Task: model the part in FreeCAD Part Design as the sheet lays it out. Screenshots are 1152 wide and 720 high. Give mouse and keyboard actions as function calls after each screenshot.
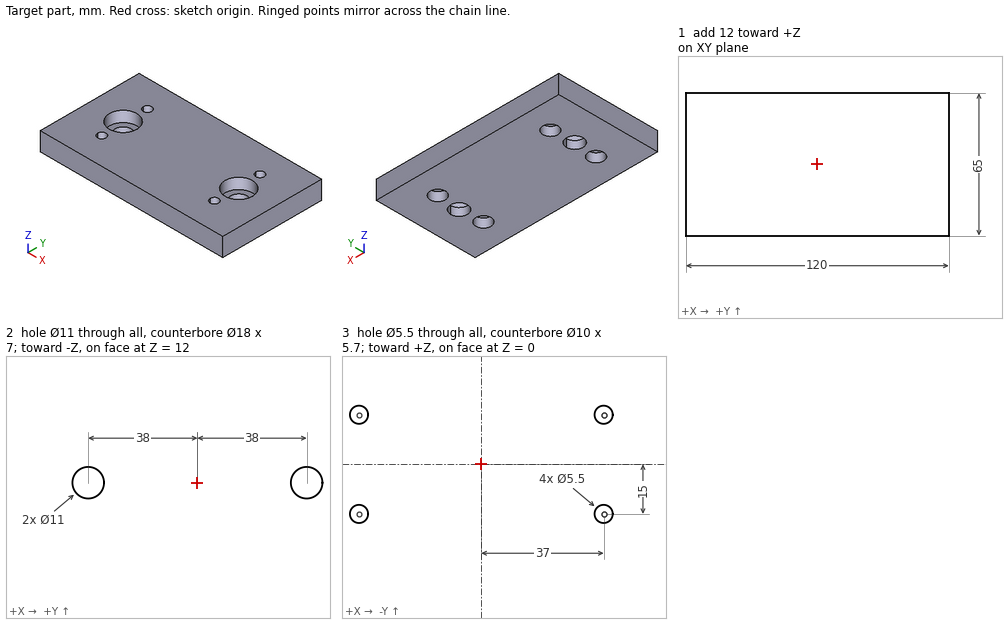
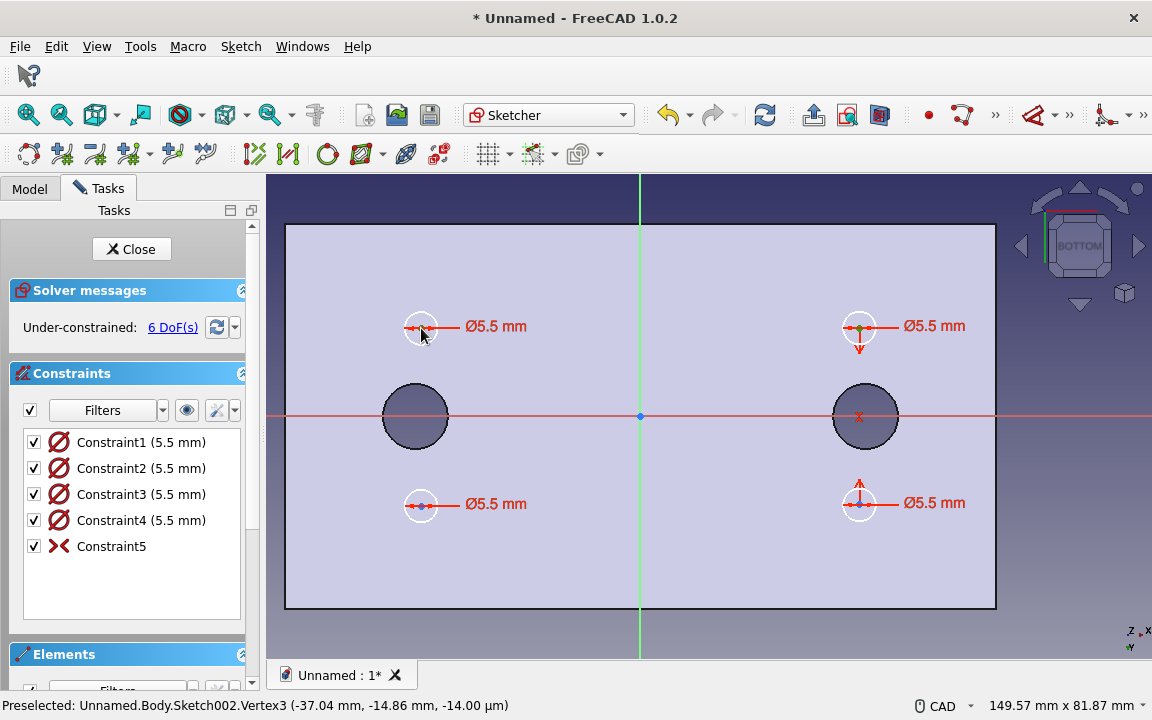
click(640, 600)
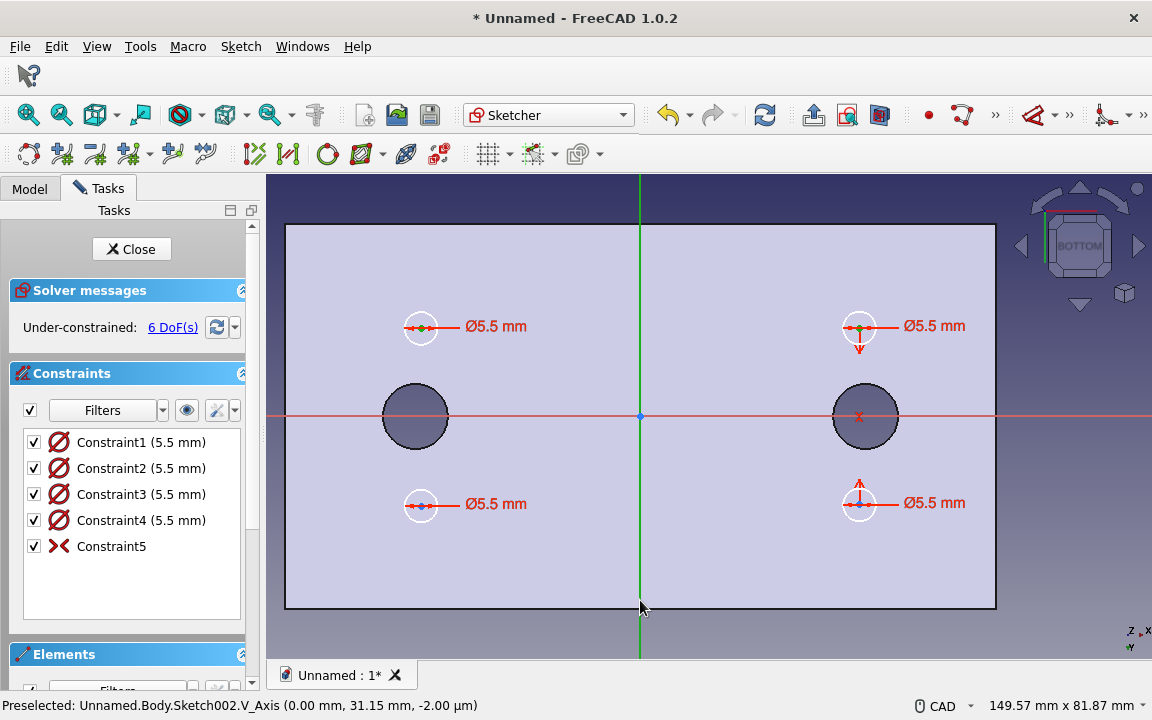
key(s)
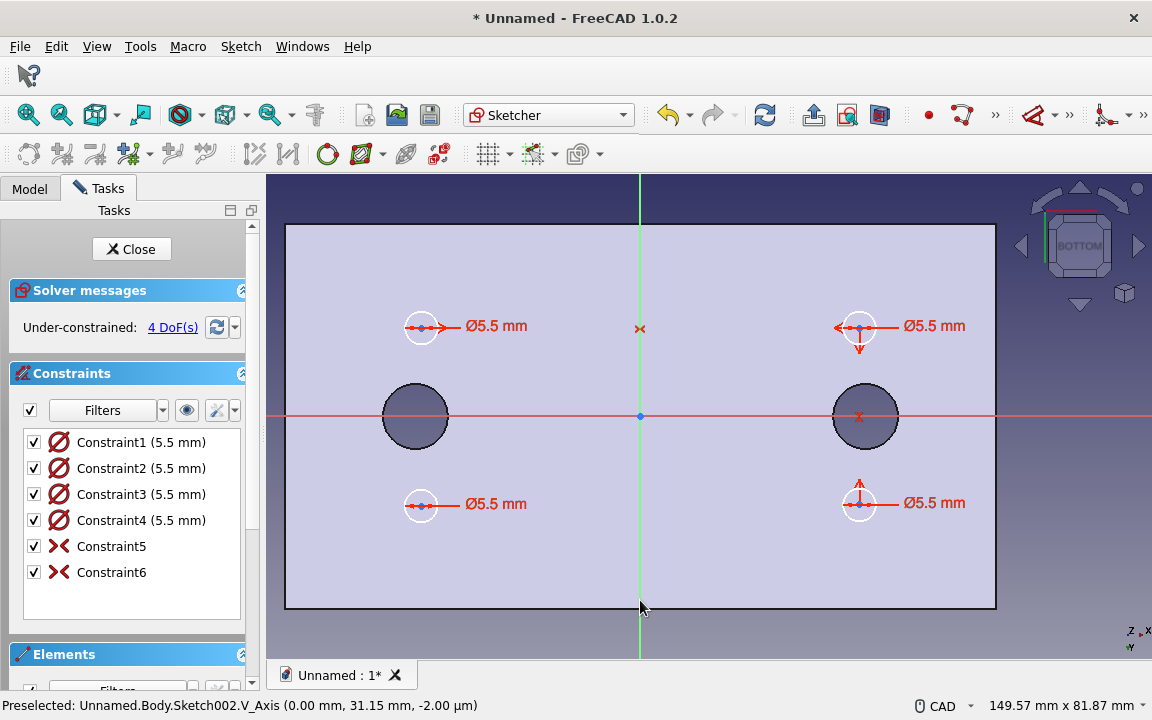
click(860, 505)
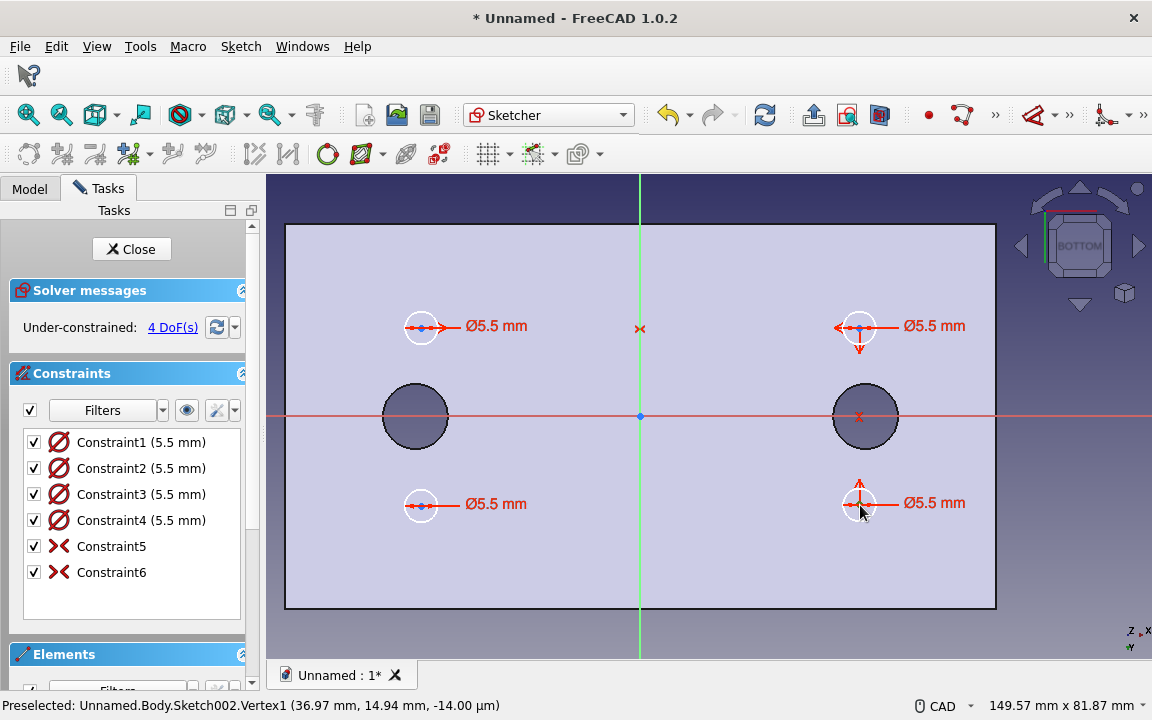
click(421, 506)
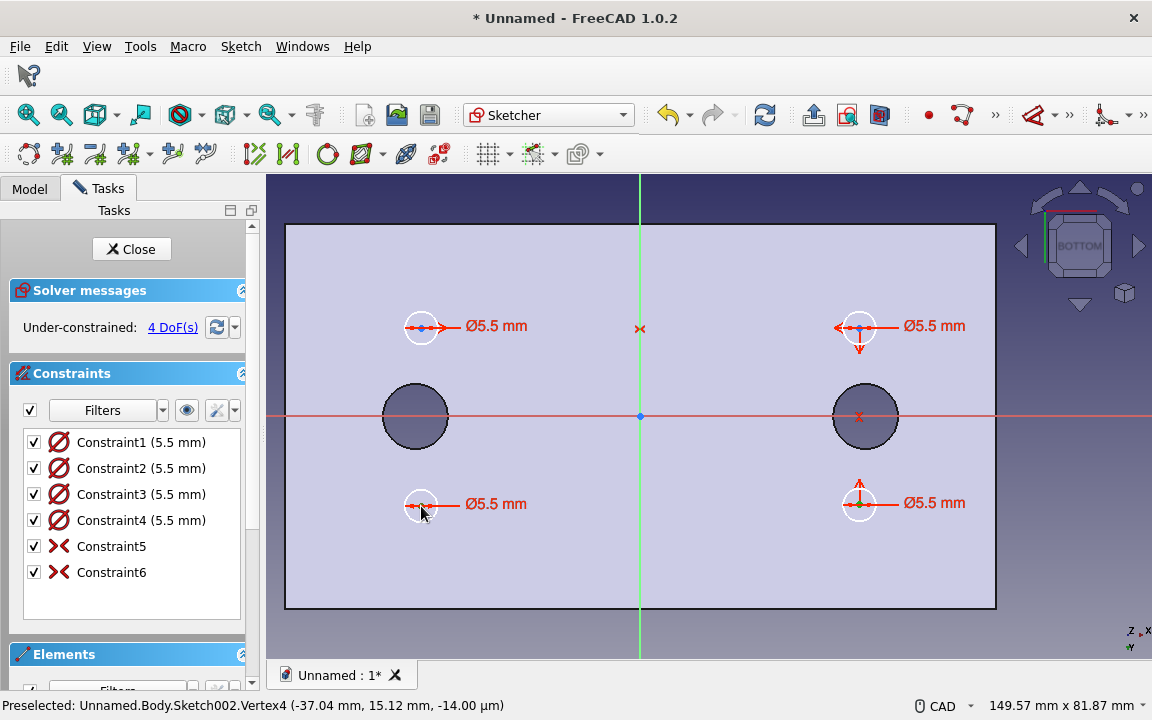
click(640, 600)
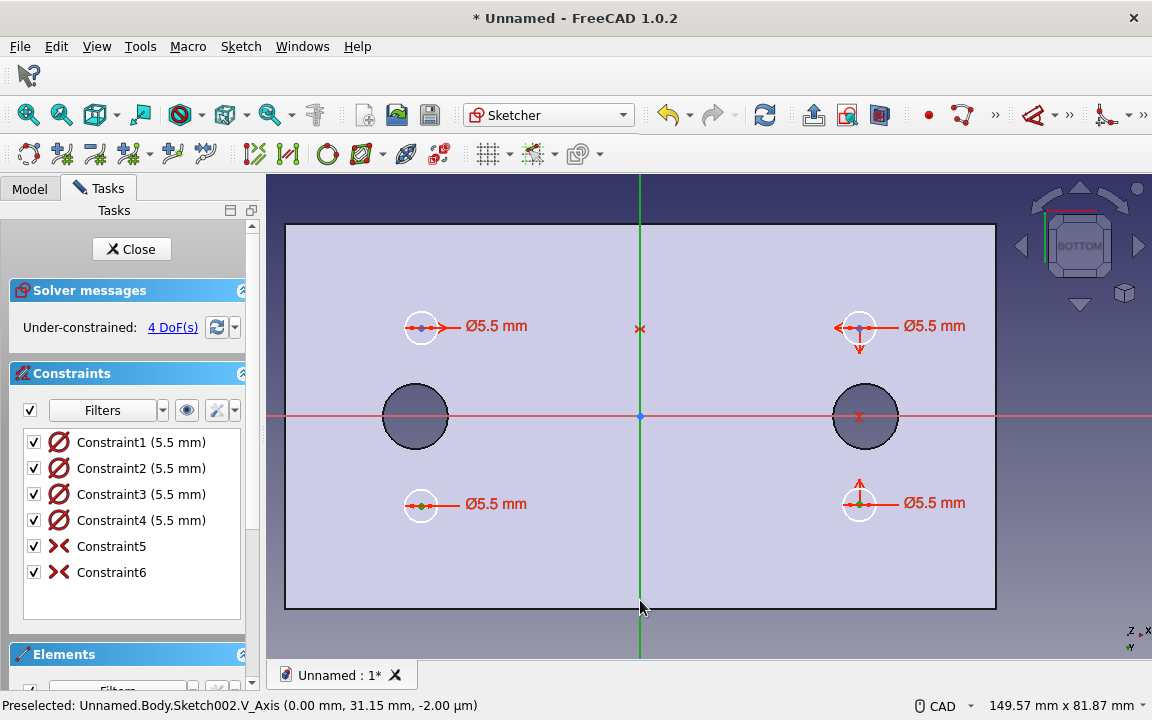
key(s)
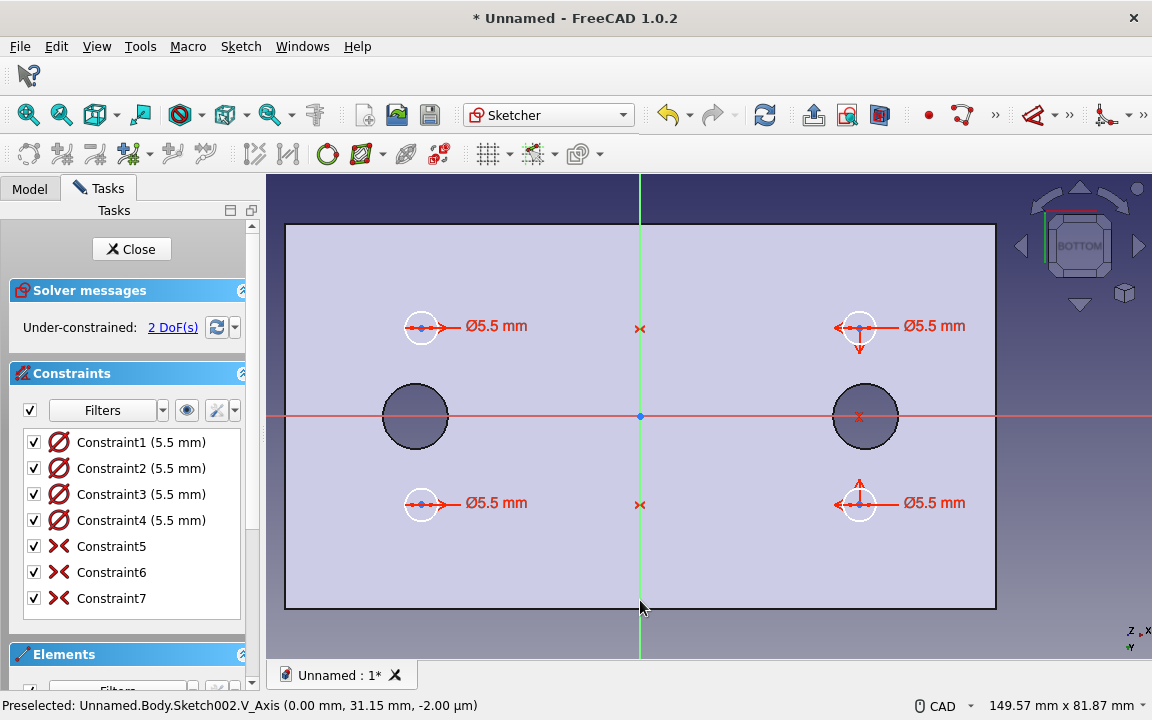
click(1032, 116)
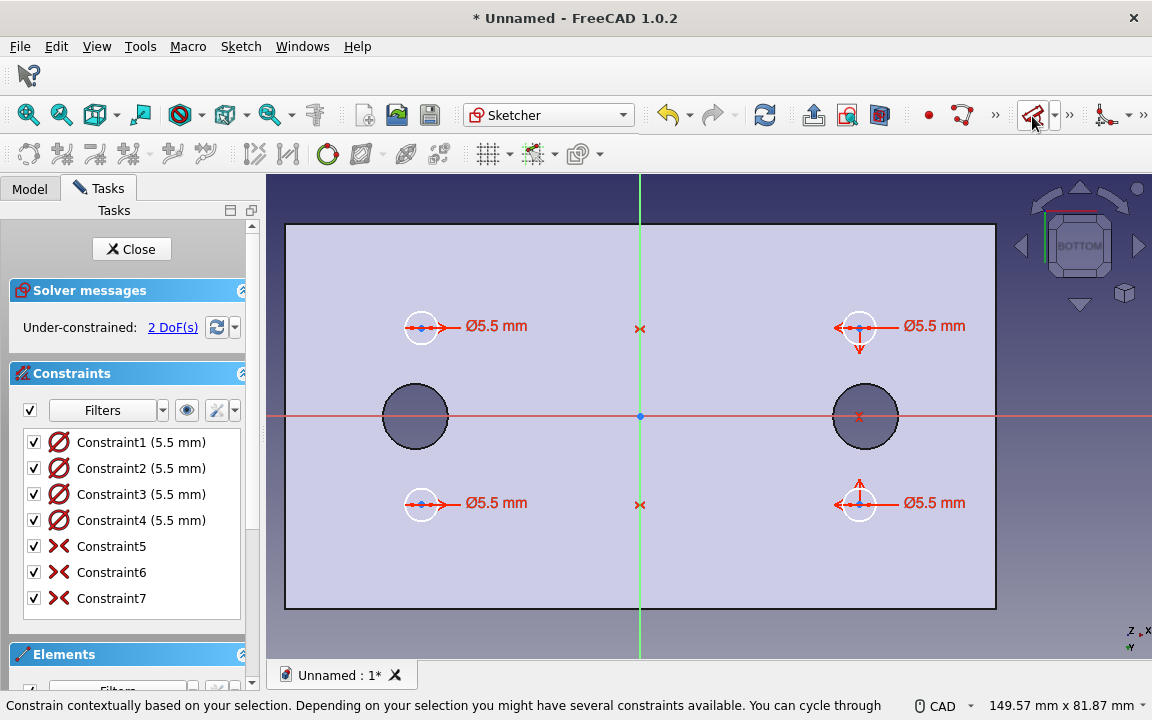
click(860, 505)
click(750, 539)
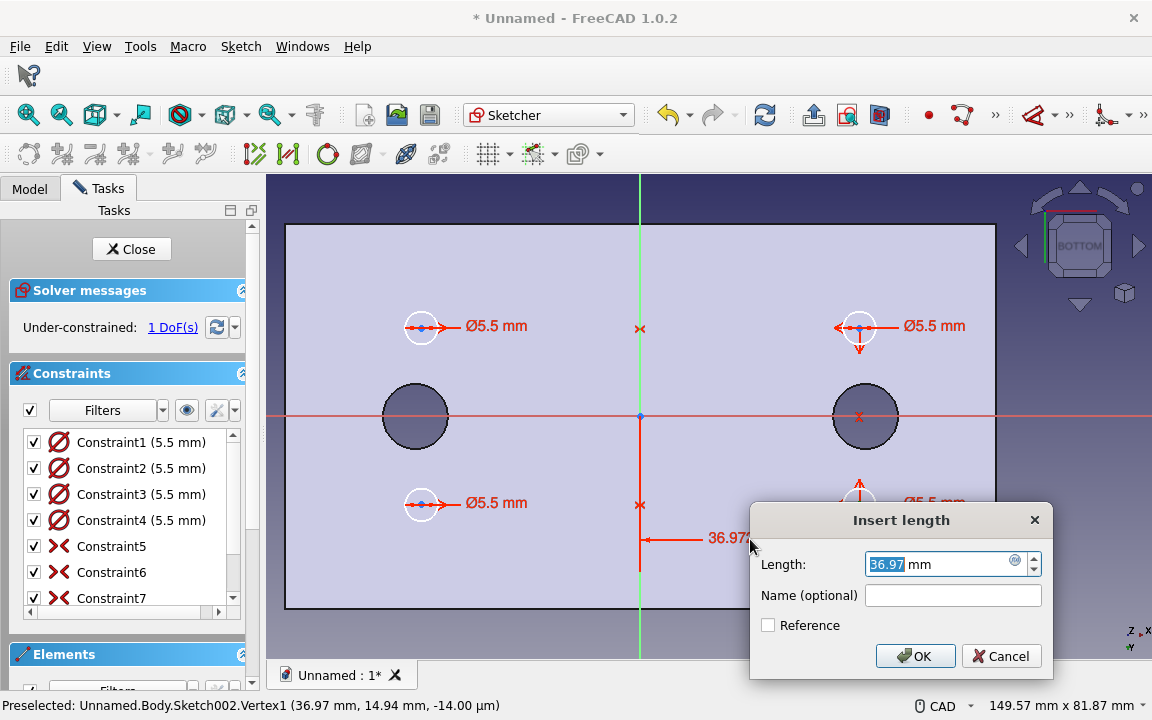
text(37)
key(Return)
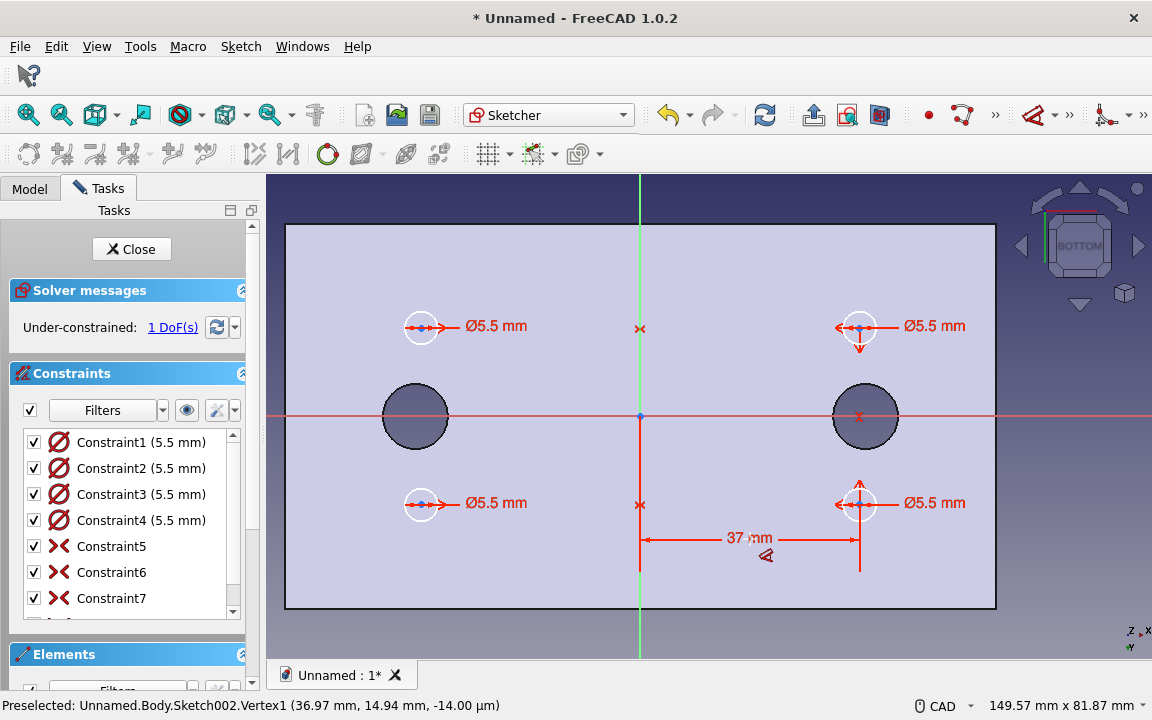
click(860, 505)
click(894, 461)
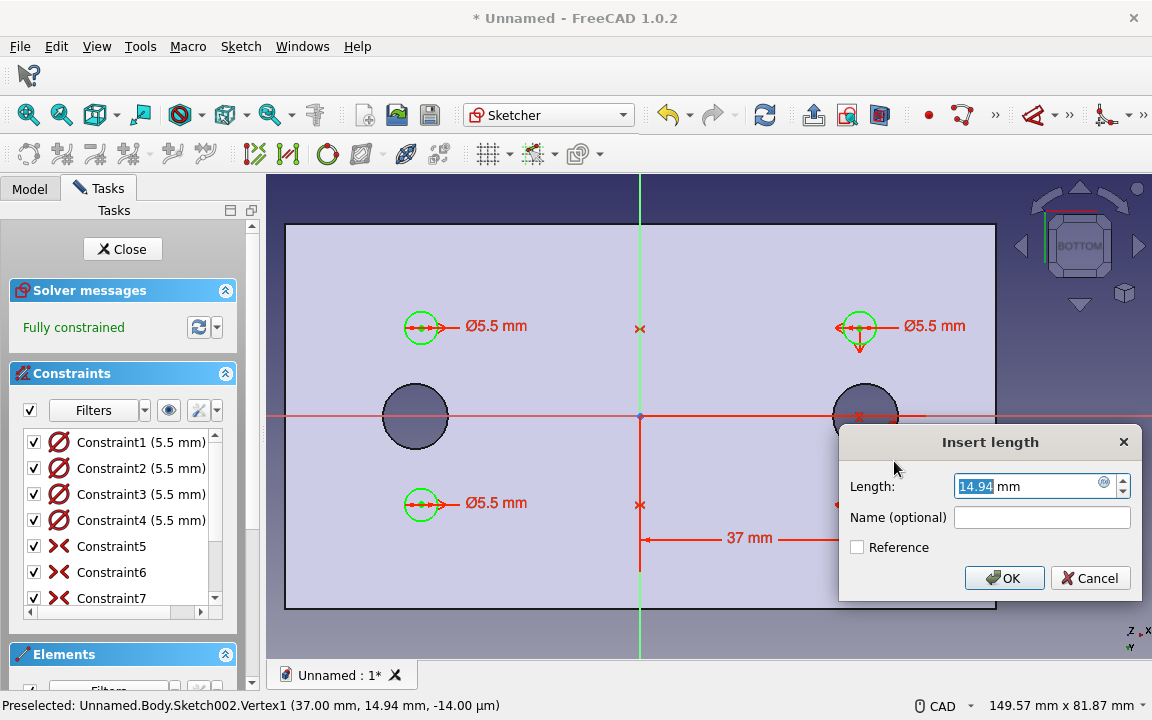
text(15)
key(Return)
key(Escape)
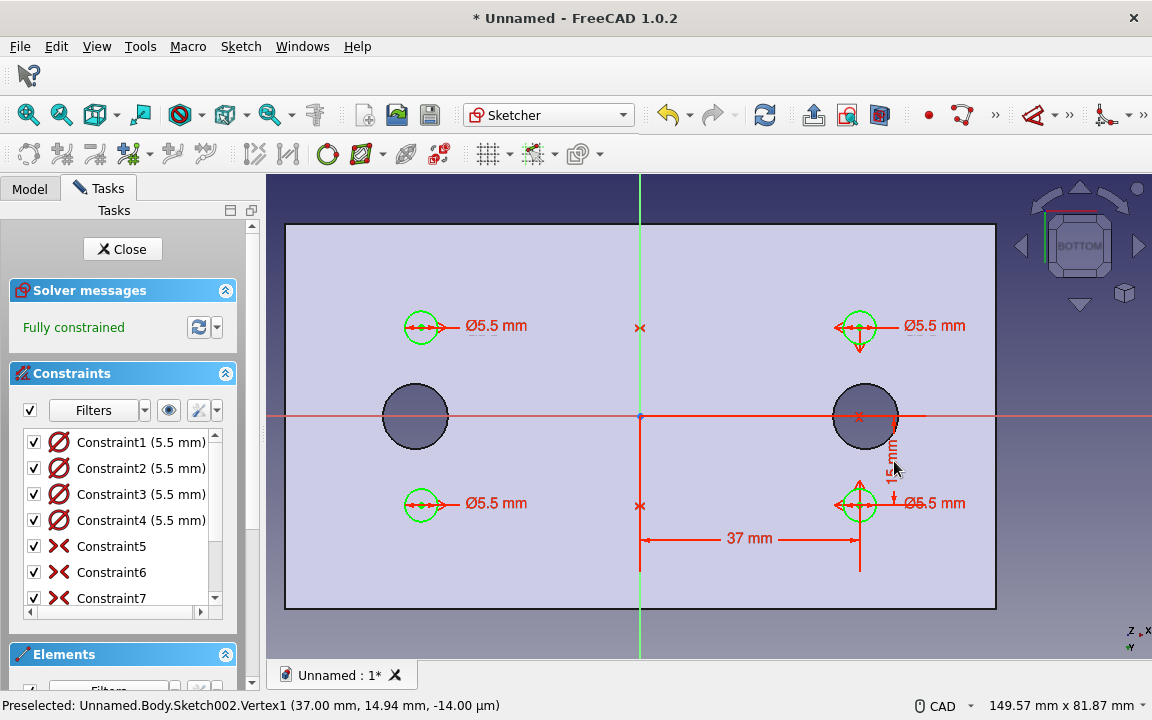
click(123, 249)